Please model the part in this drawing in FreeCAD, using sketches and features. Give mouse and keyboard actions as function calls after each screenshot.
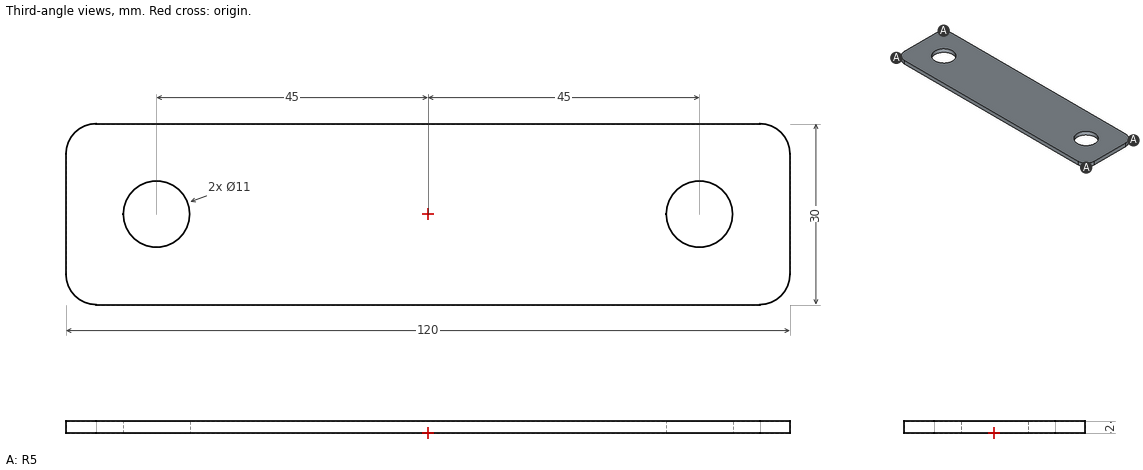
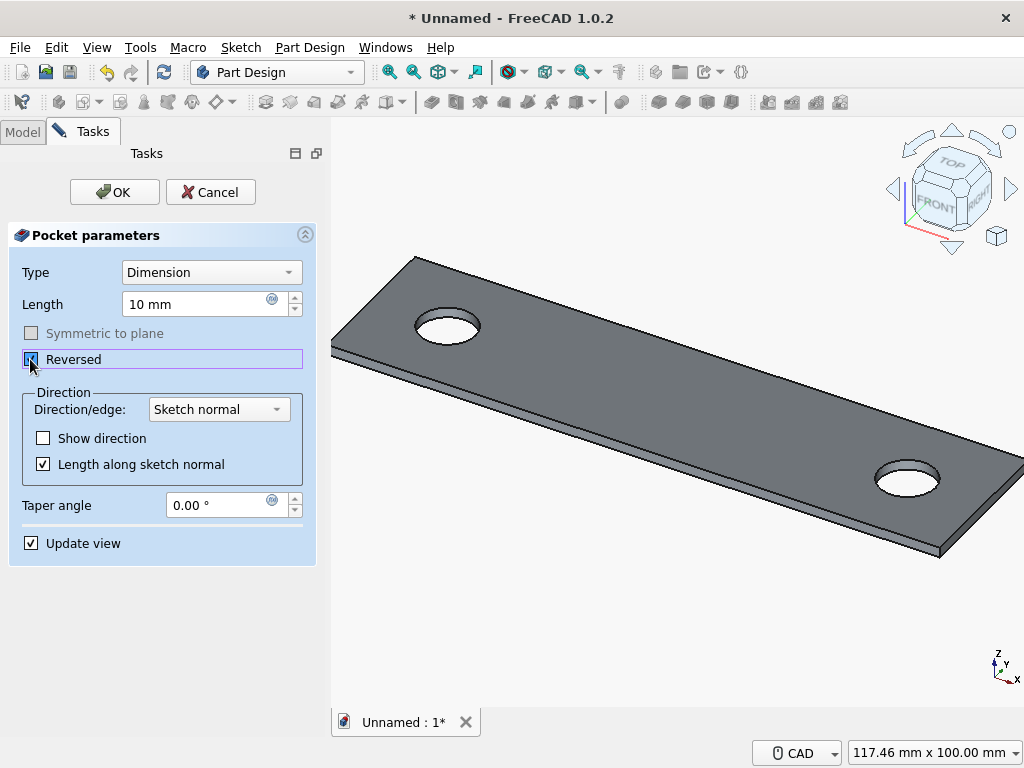
click(115, 192)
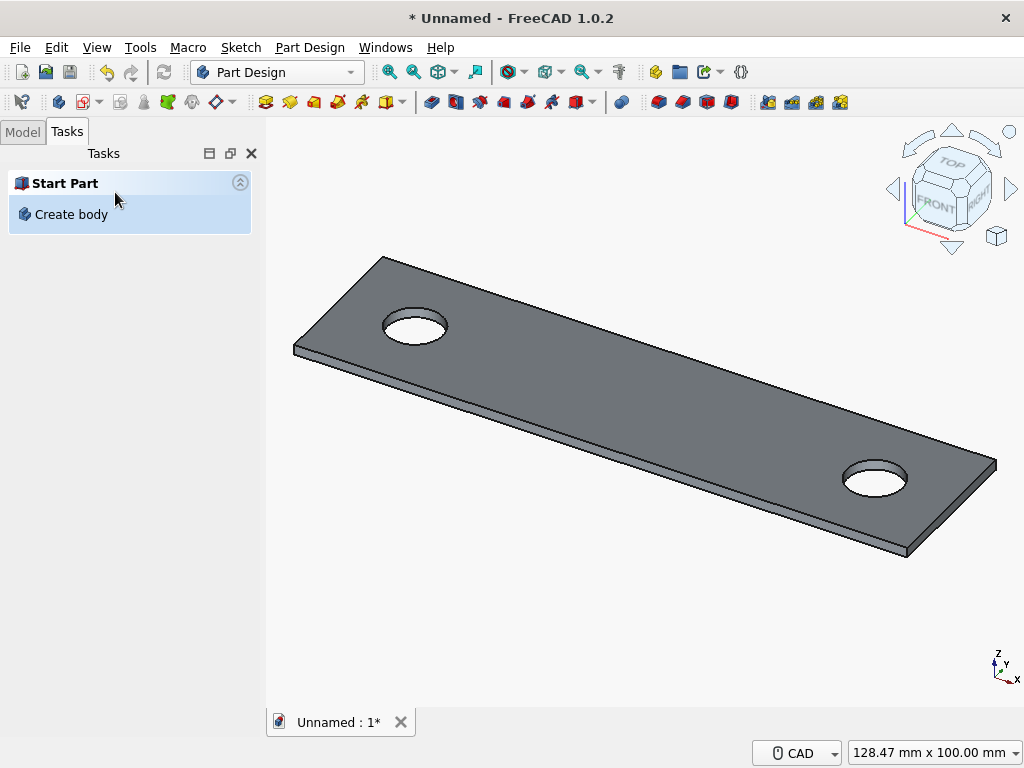
click(907, 553)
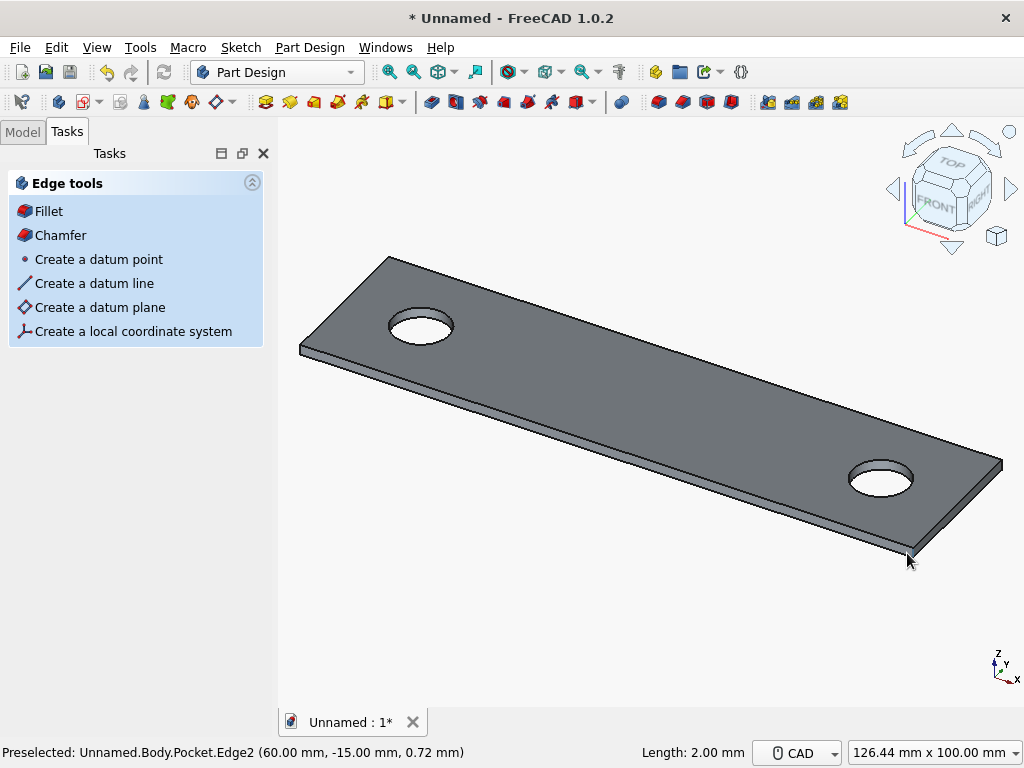
key(0)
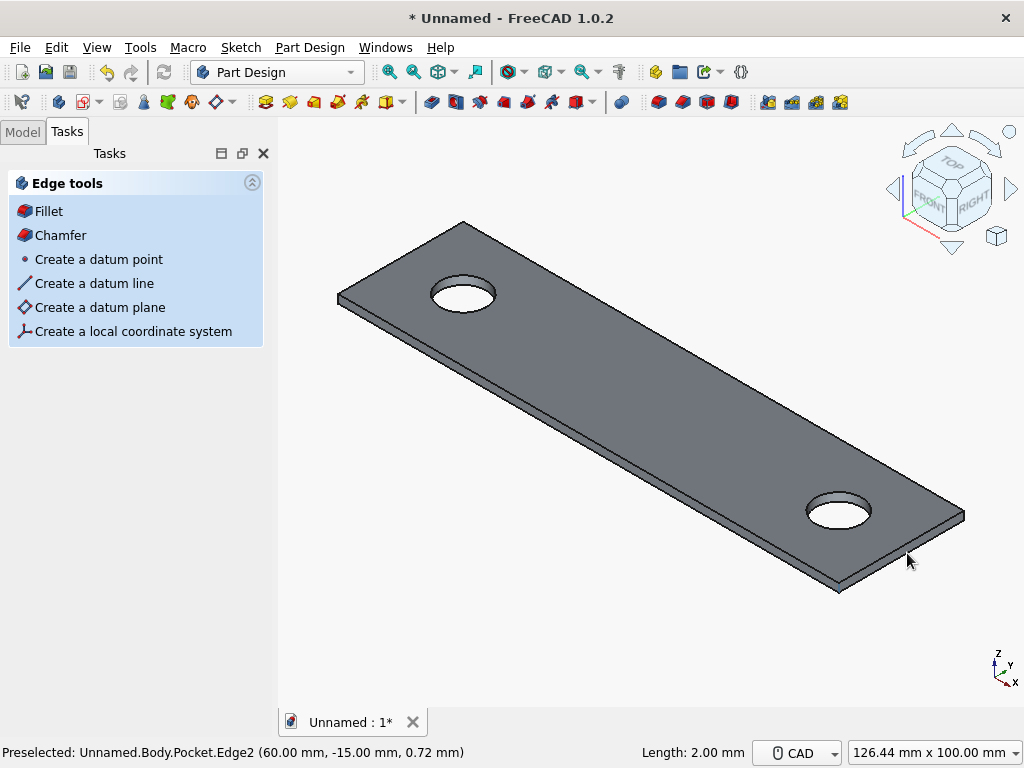
scroll(338, 298, up, 7)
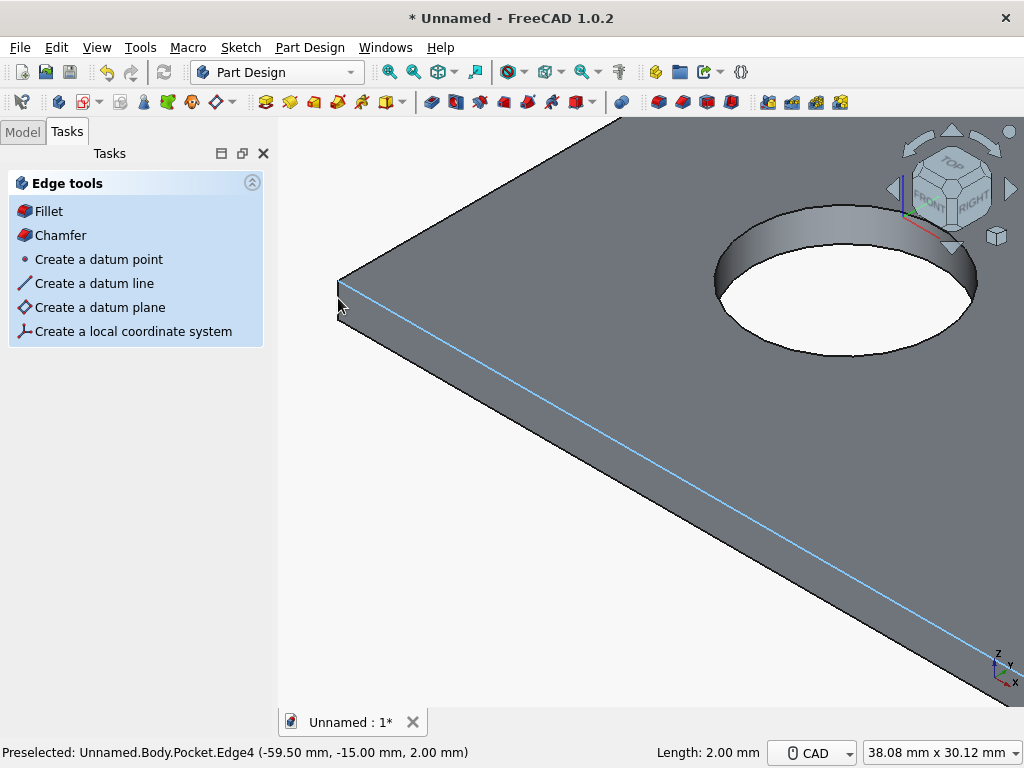
click(390, 72)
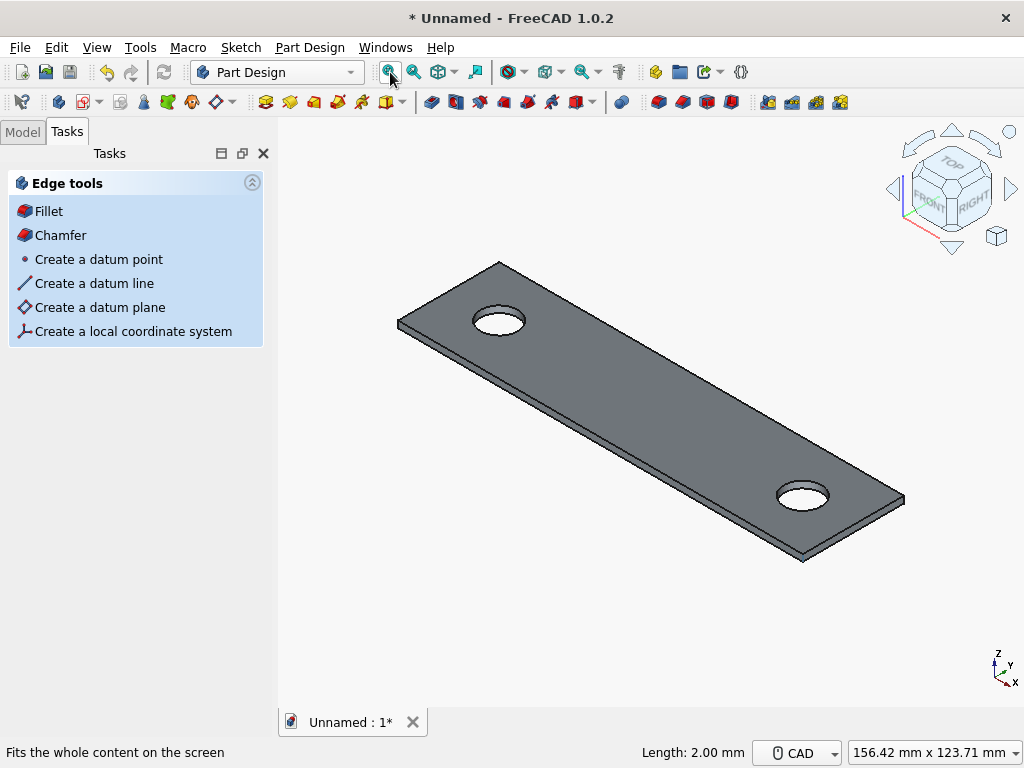
key(2)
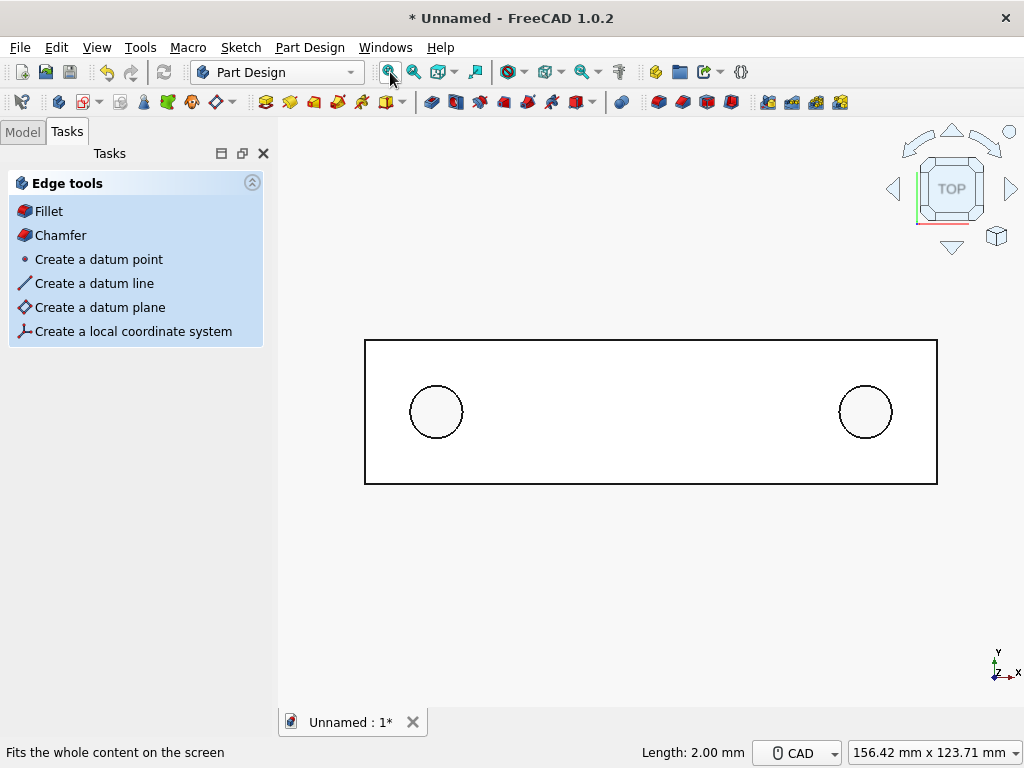
scroll(365, 483, up, 8)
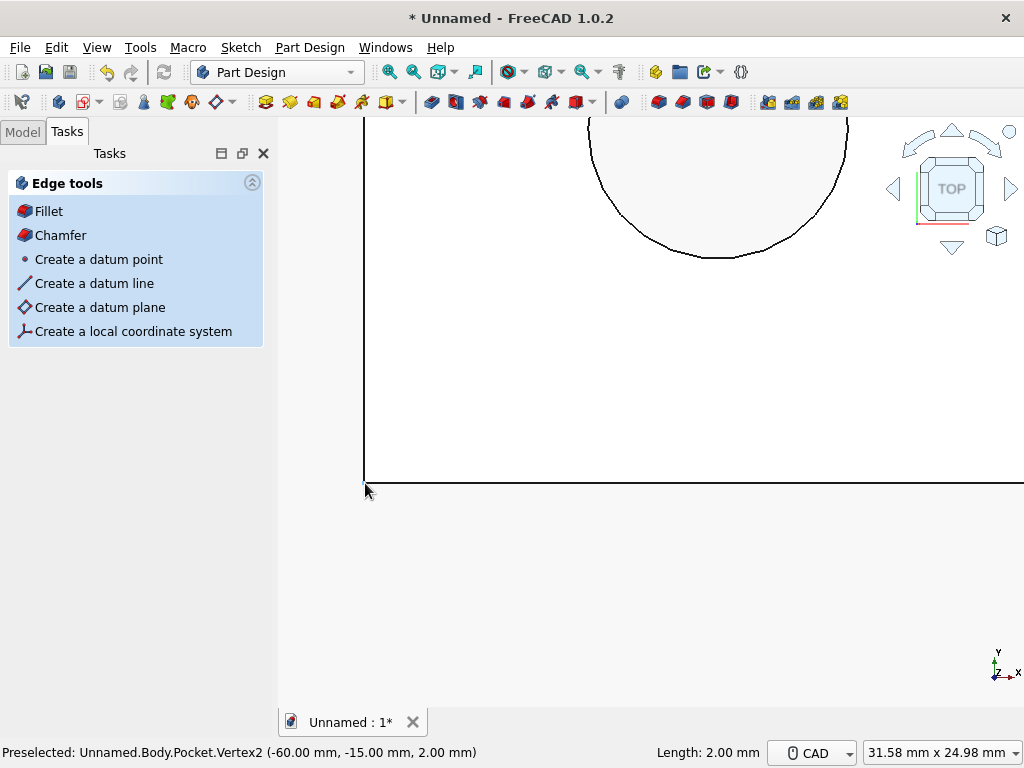
click(390, 72)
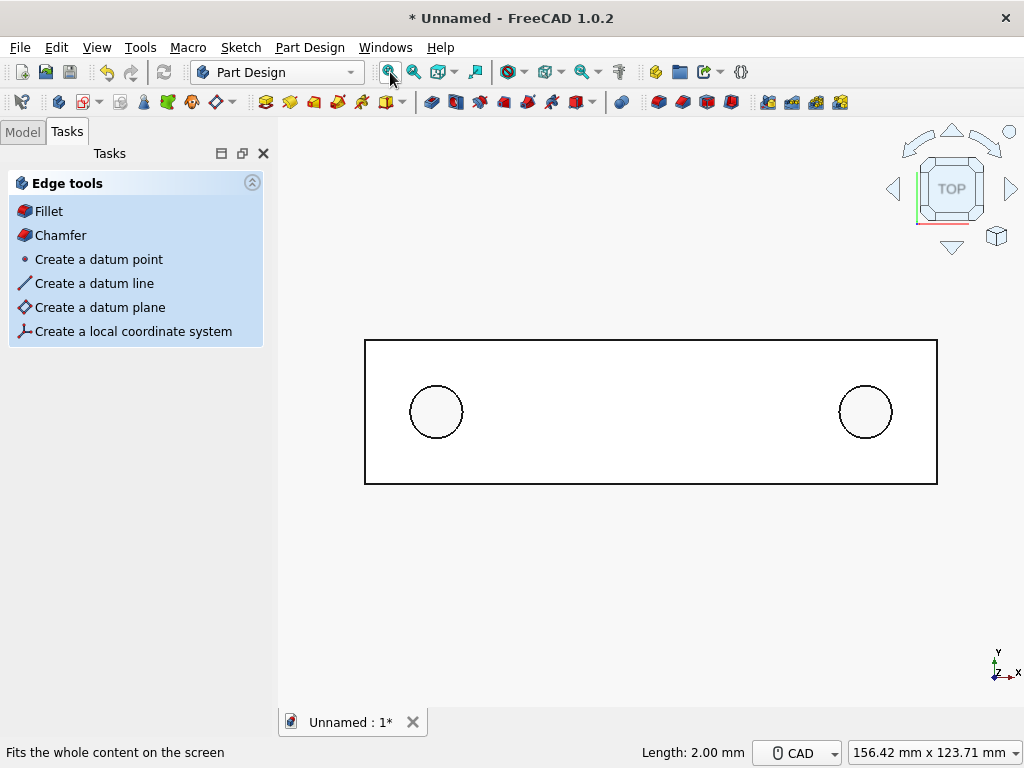
key(1)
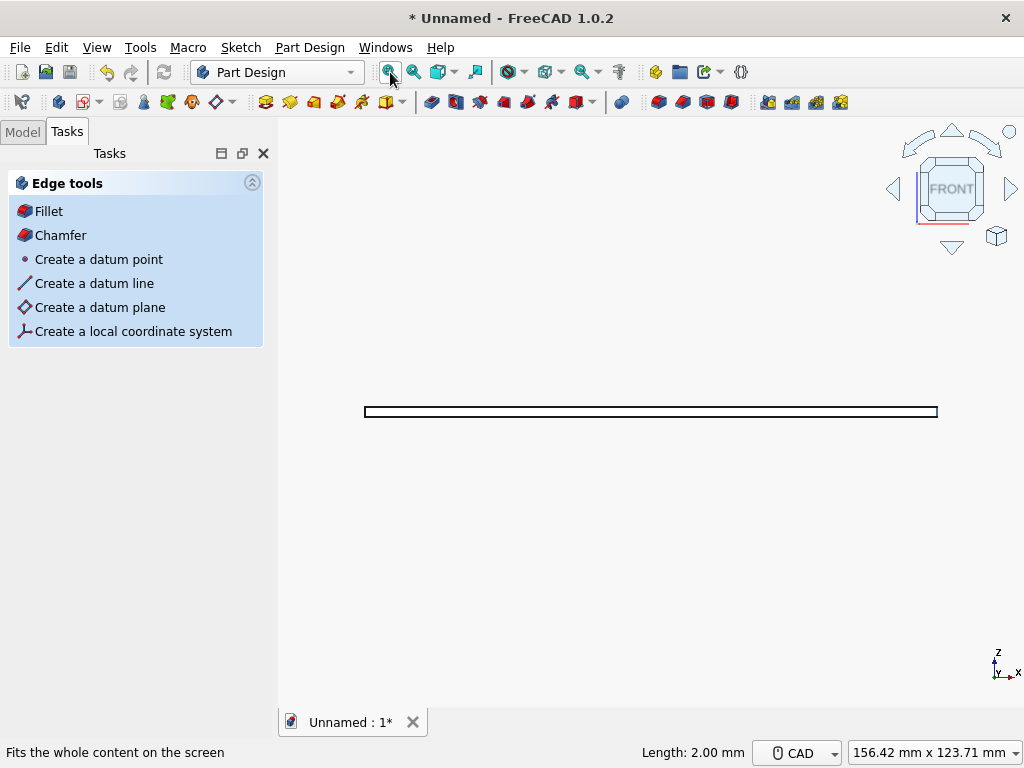
scroll(365, 411, up, 8)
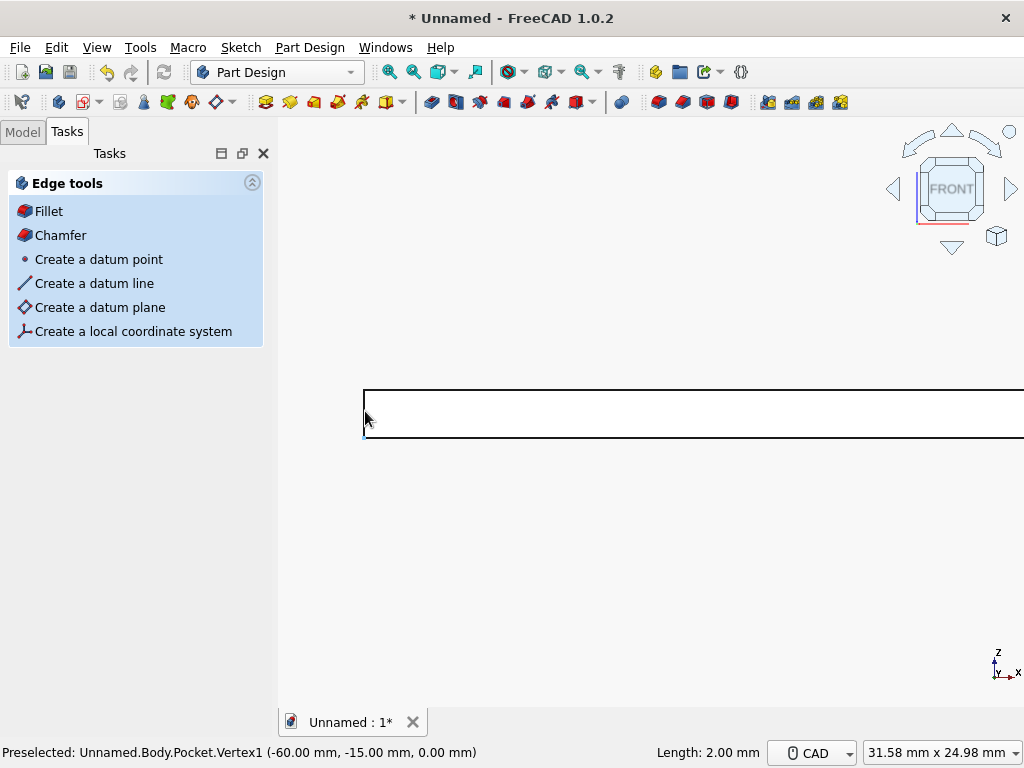
click(364, 413, ctrl)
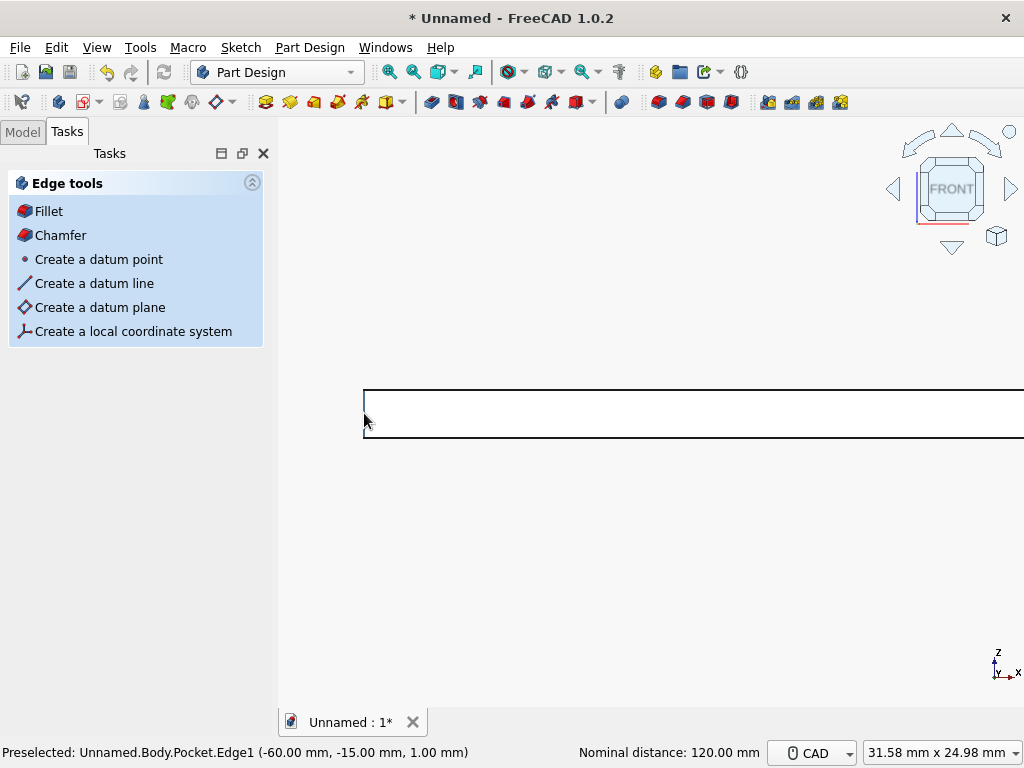
key(v)
key(f)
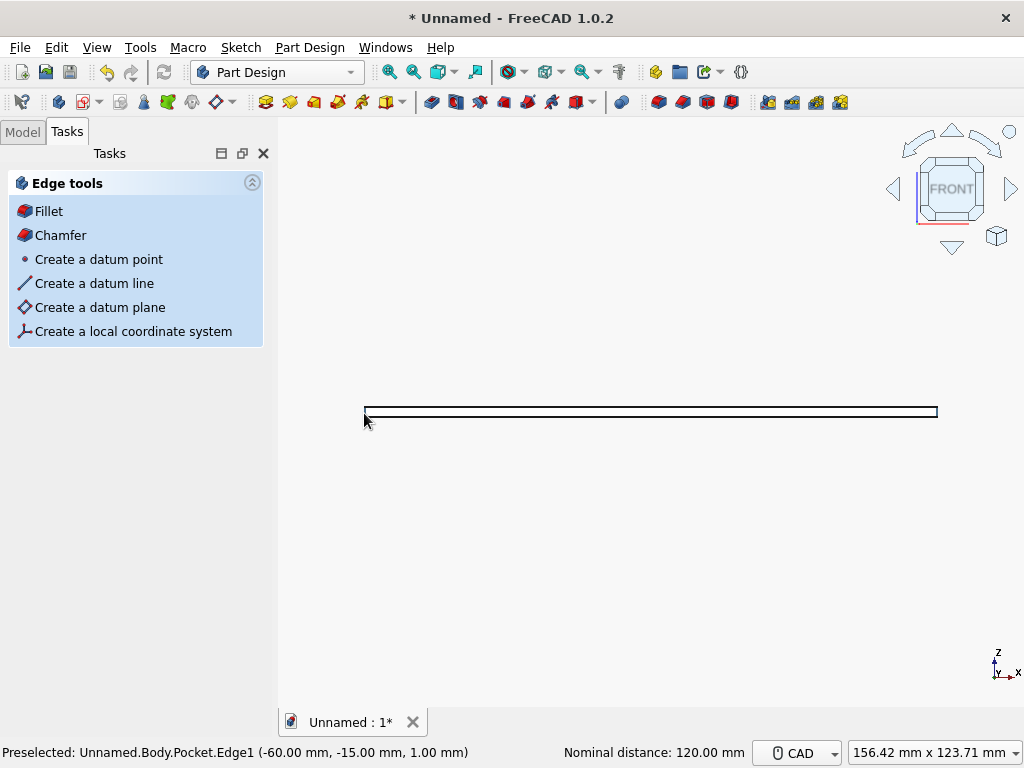
key(3)